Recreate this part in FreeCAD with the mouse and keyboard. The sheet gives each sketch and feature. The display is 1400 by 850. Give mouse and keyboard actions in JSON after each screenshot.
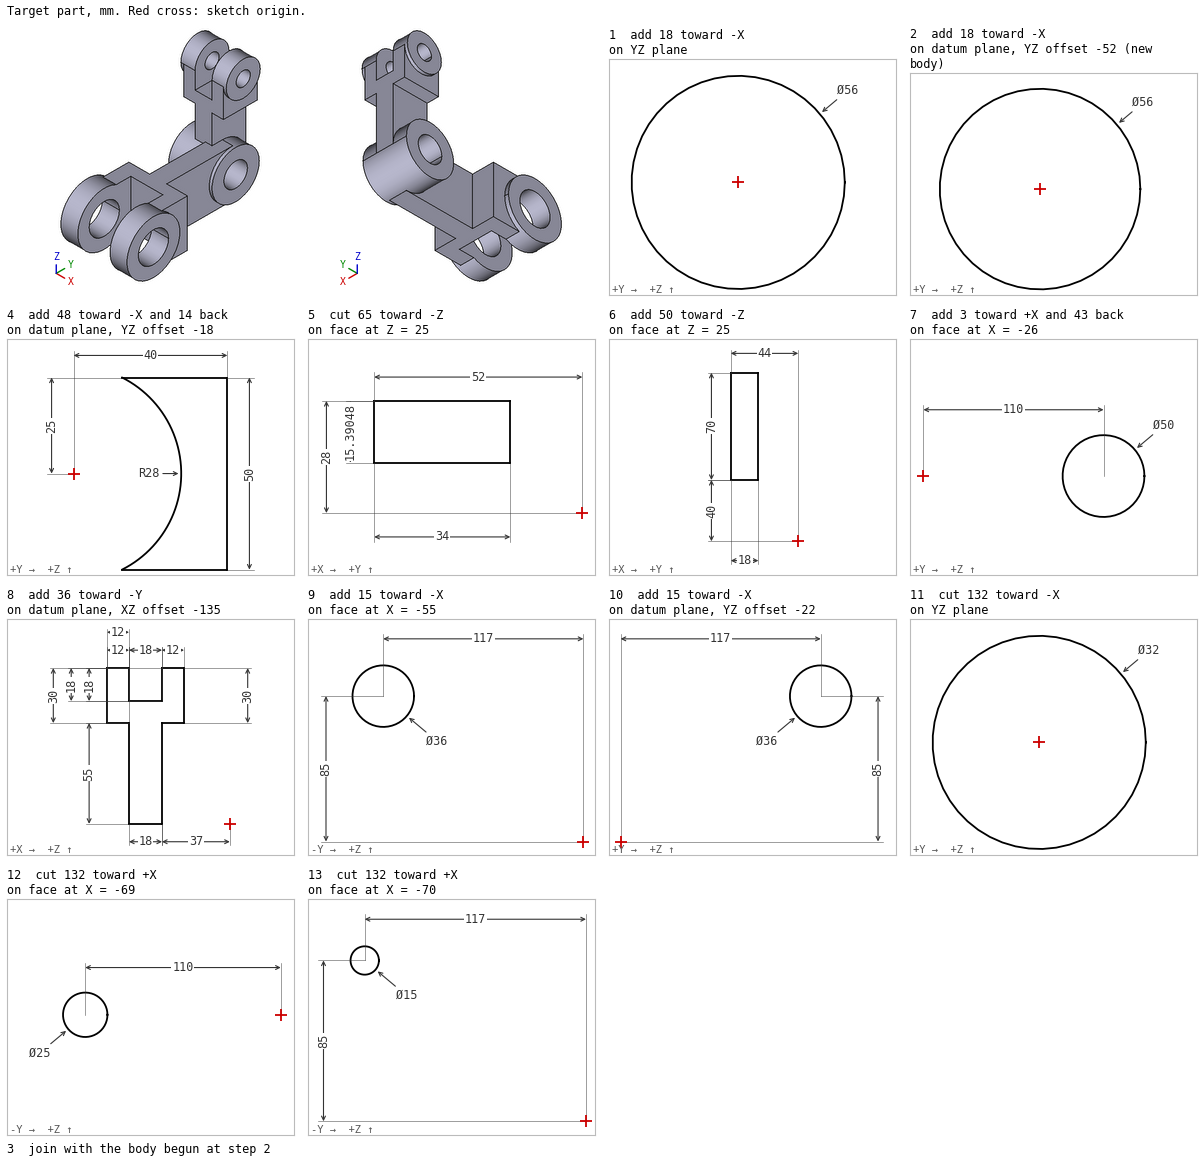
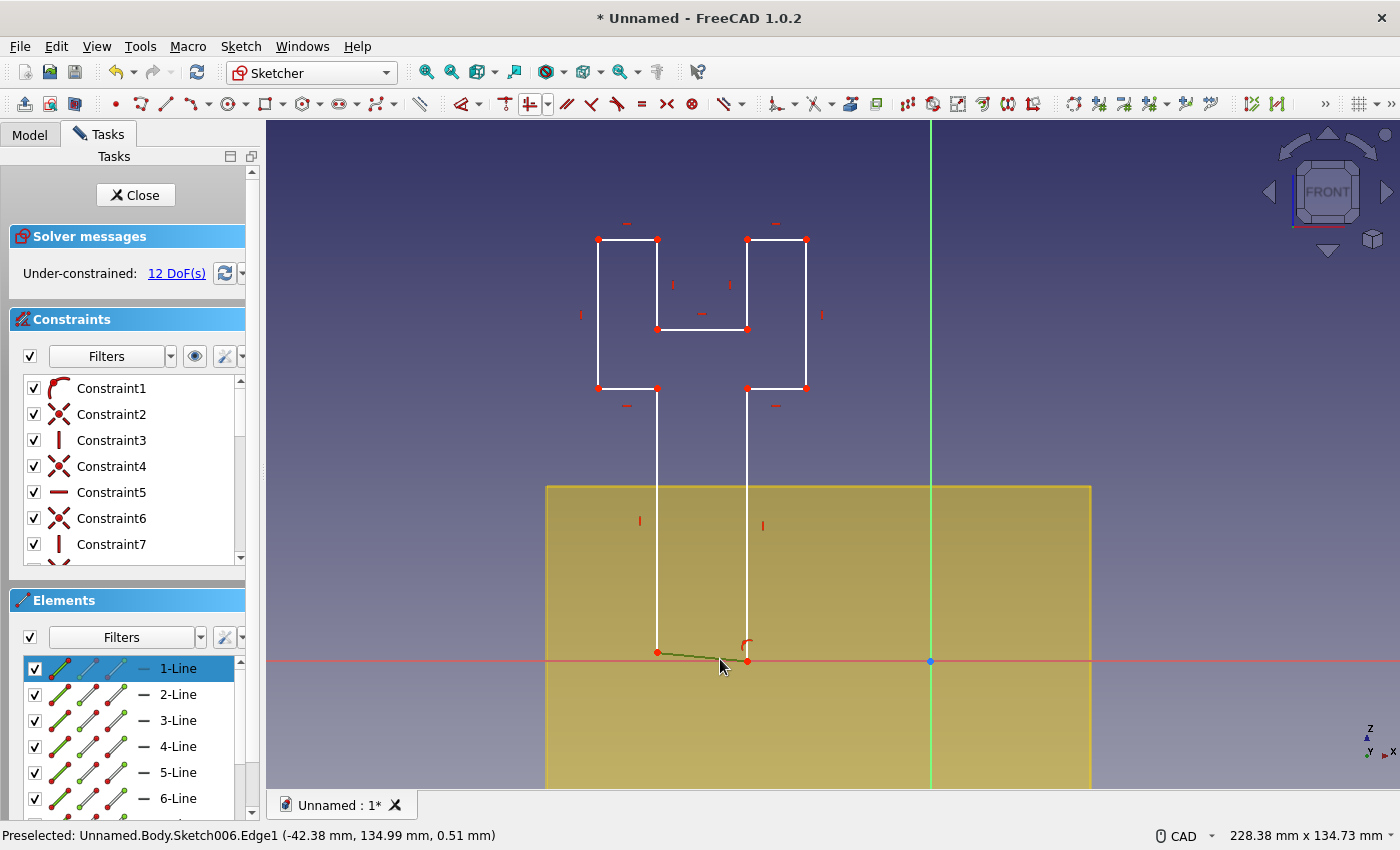
{"action": "key", "text": "h"}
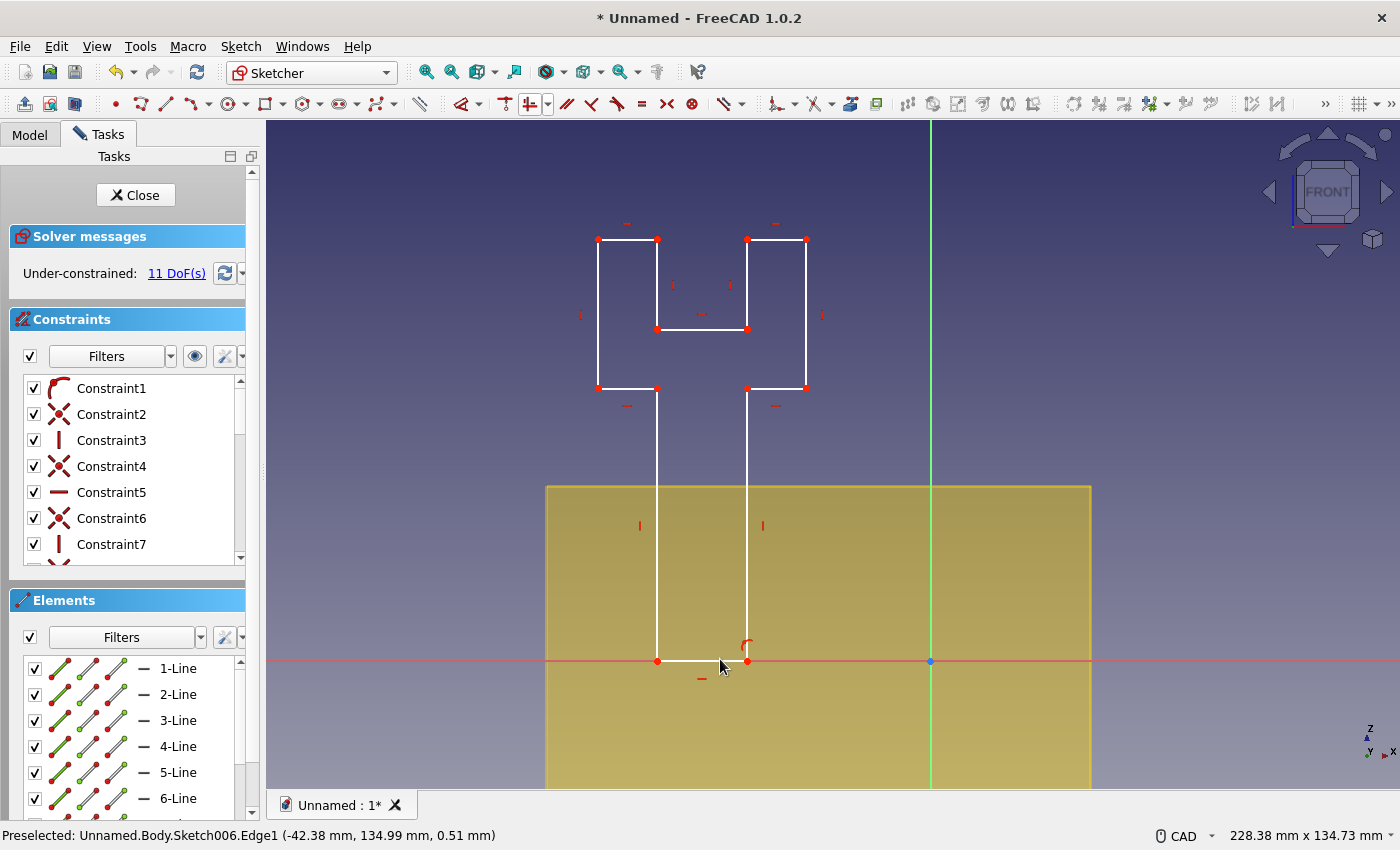
{"action": "left_click", "coordinate": [720, 661]}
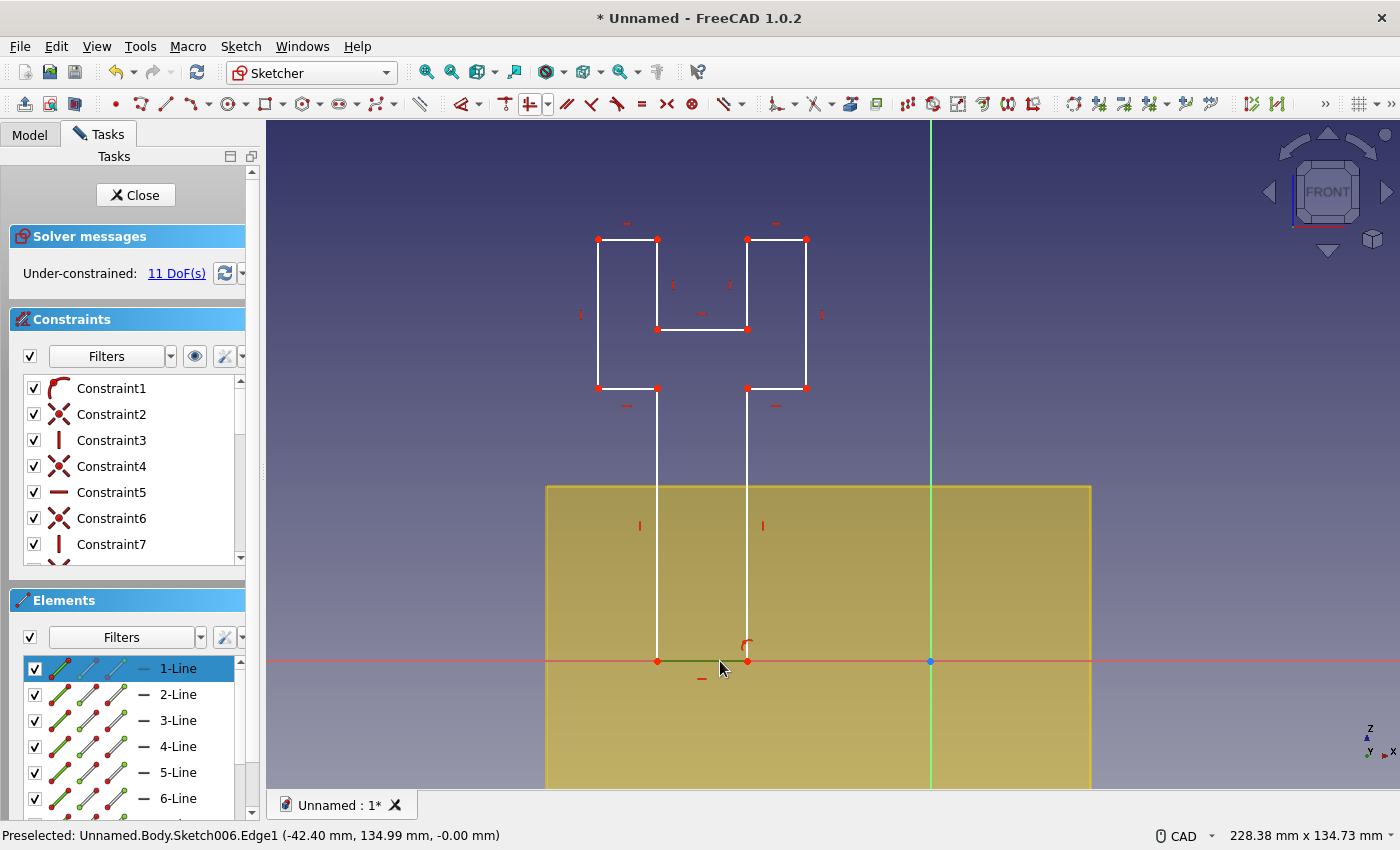
{"action": "key", "text": "l"}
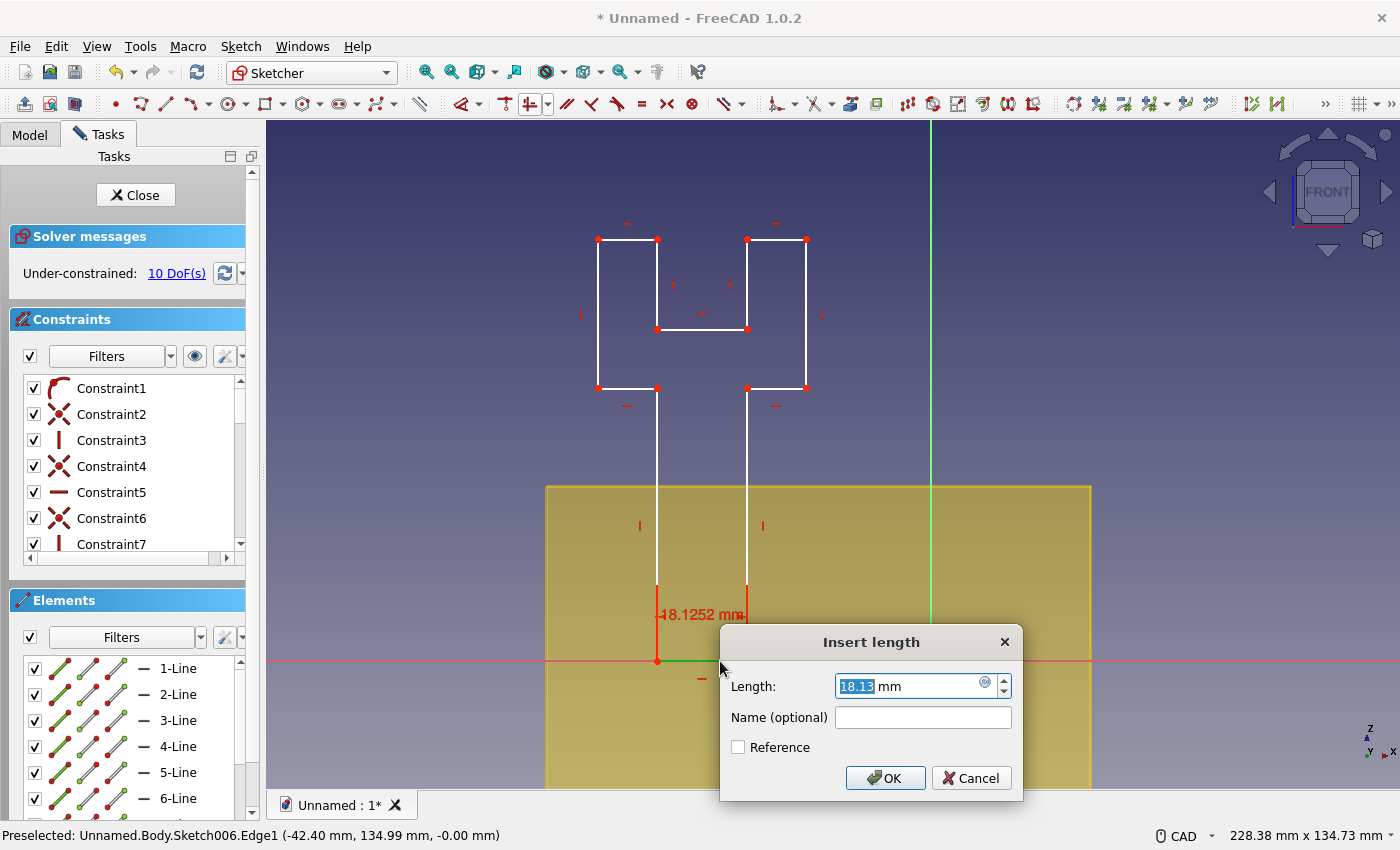
{"action": "type", "text": "18"}
{"action": "key", "text": "Return"}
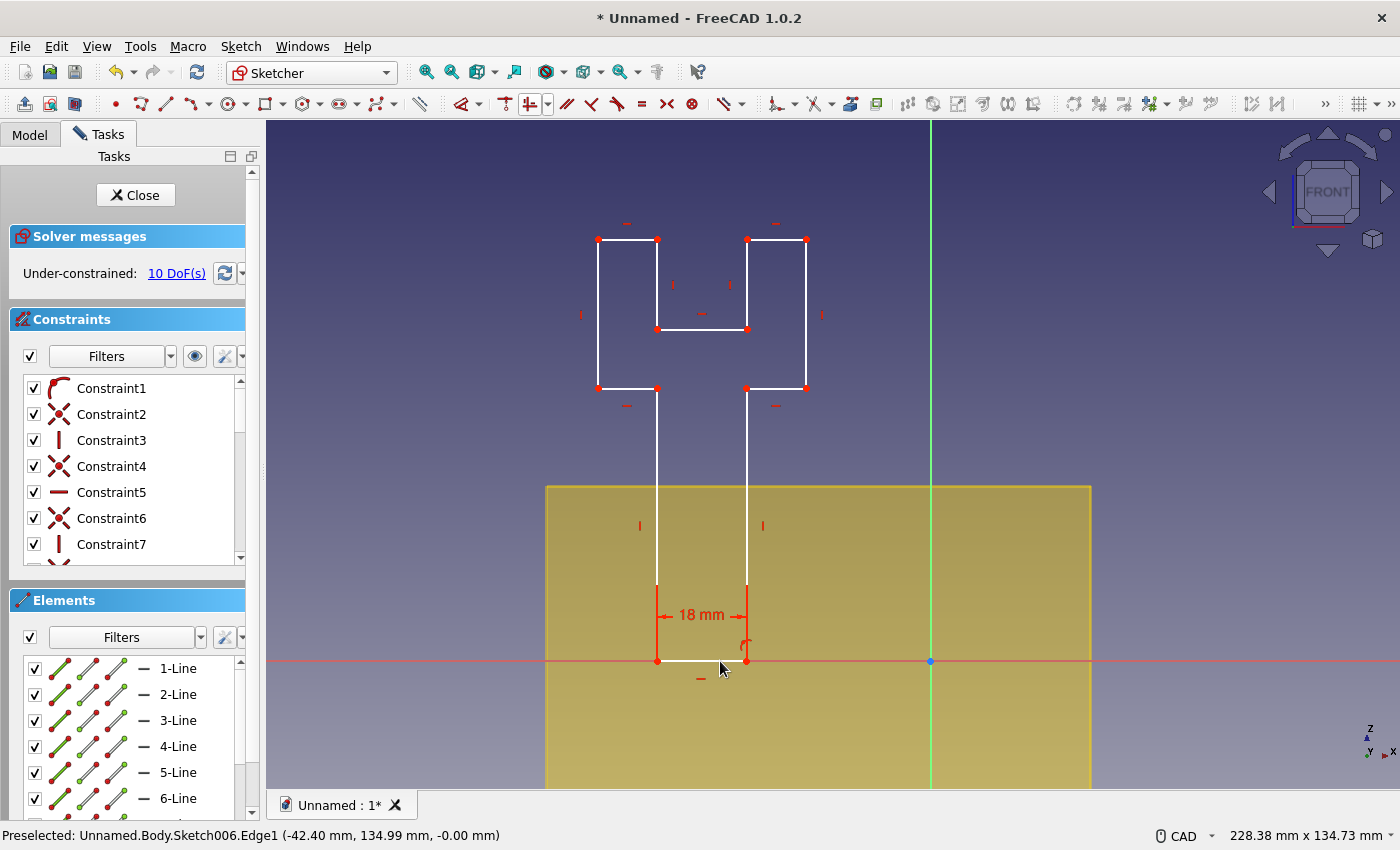
{"action": "left_click", "coordinate": [657, 580]}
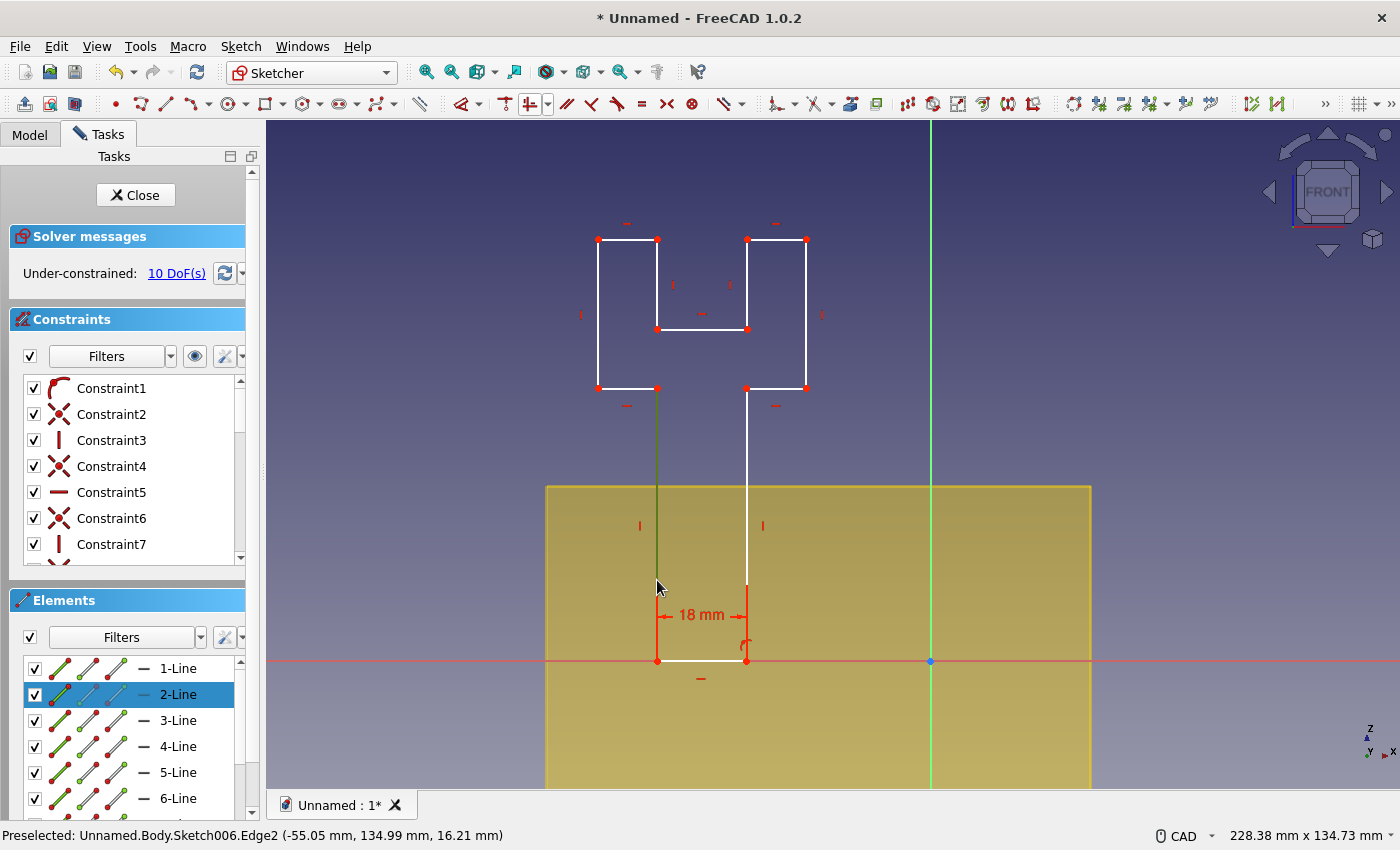
{"action": "key", "text": "i"}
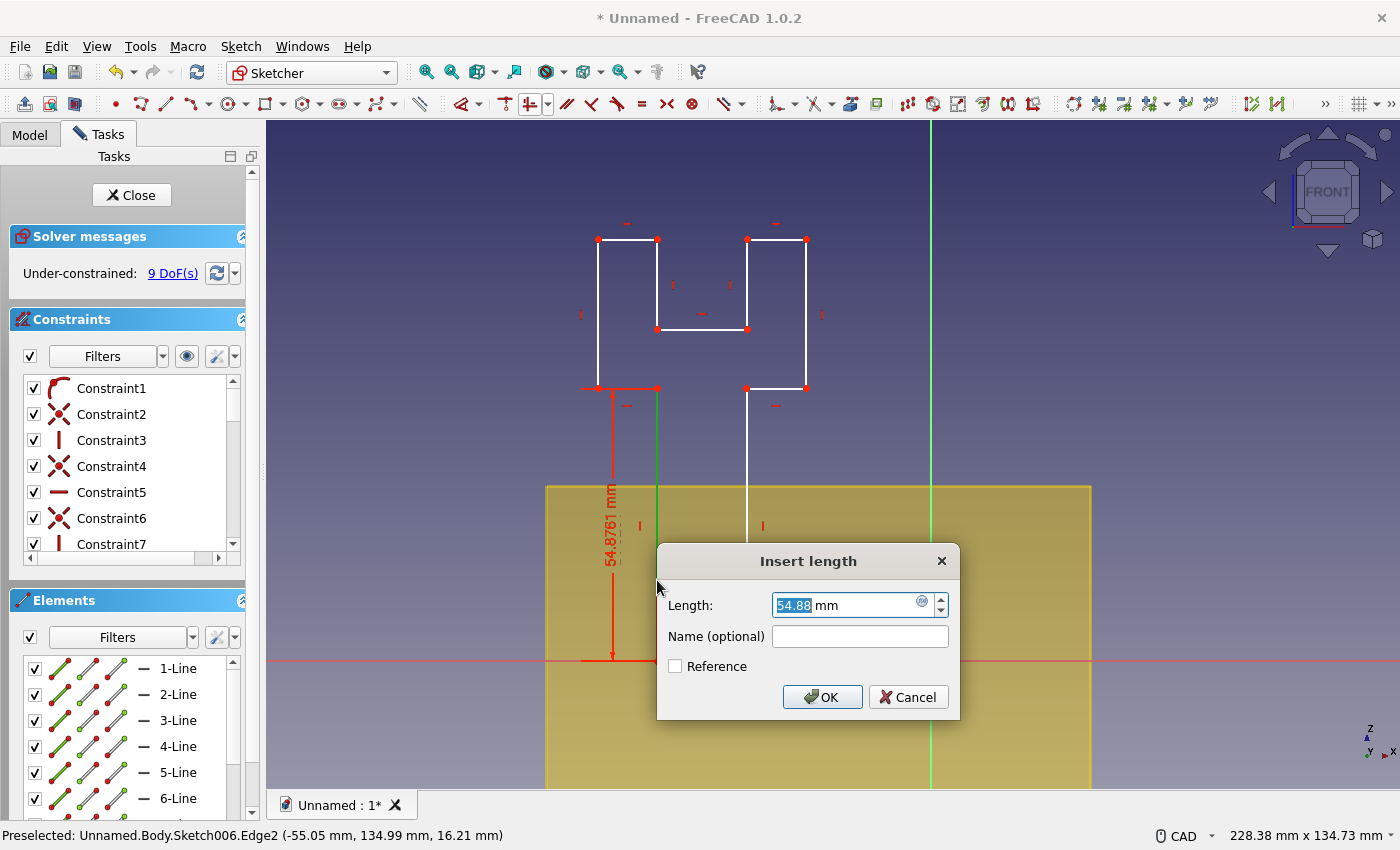
{"action": "type", "text": "55"}
{"action": "key", "text": "Return"}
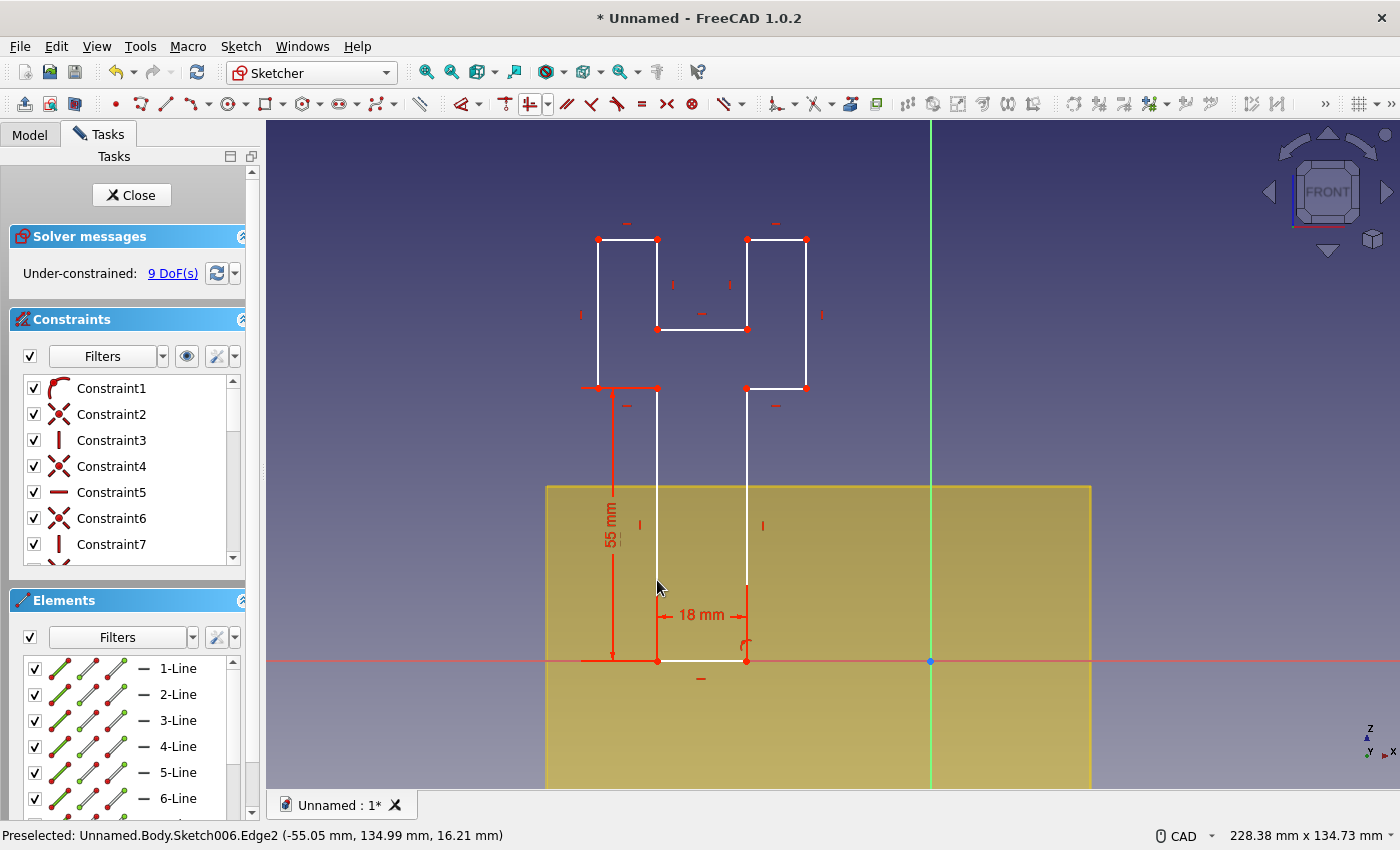
{"action": "left_click", "coordinate": [639, 388]}